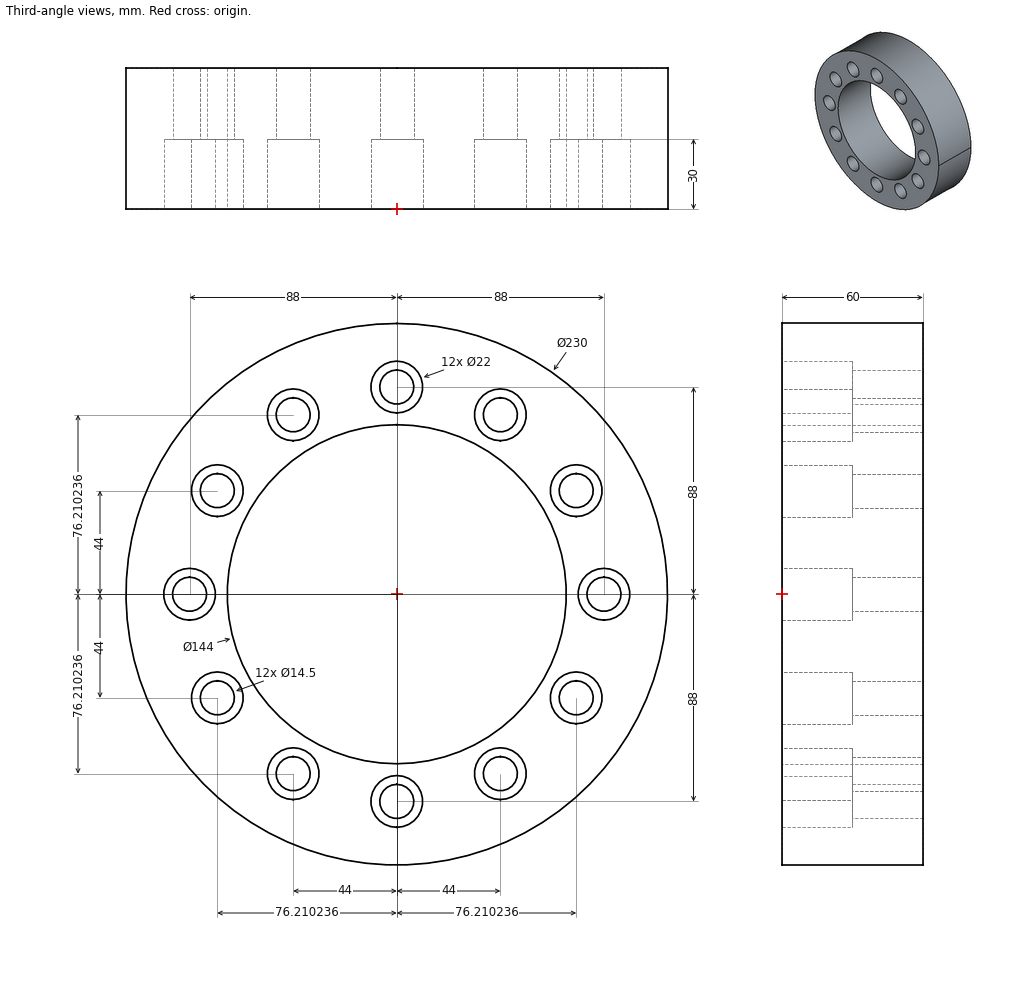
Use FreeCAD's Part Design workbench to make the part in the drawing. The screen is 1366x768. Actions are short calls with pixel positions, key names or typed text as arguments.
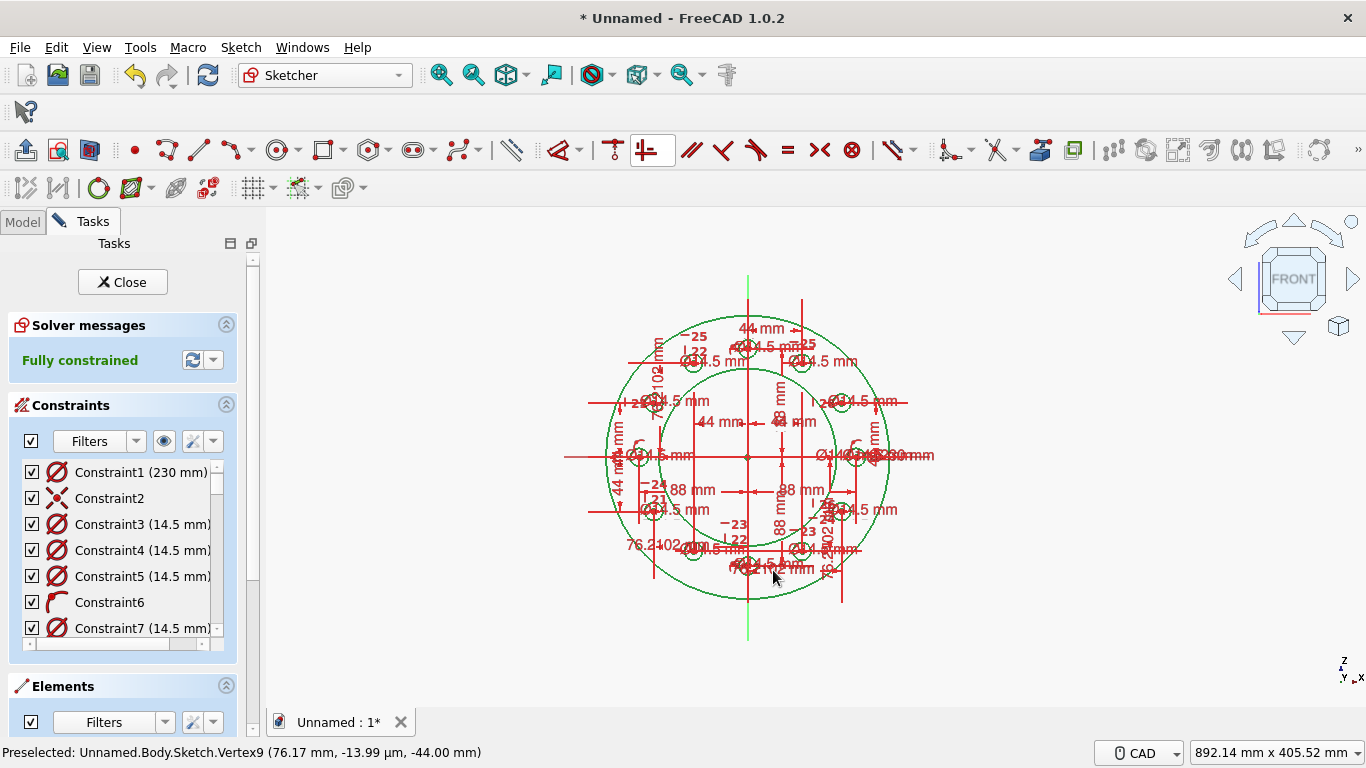
click(123, 282)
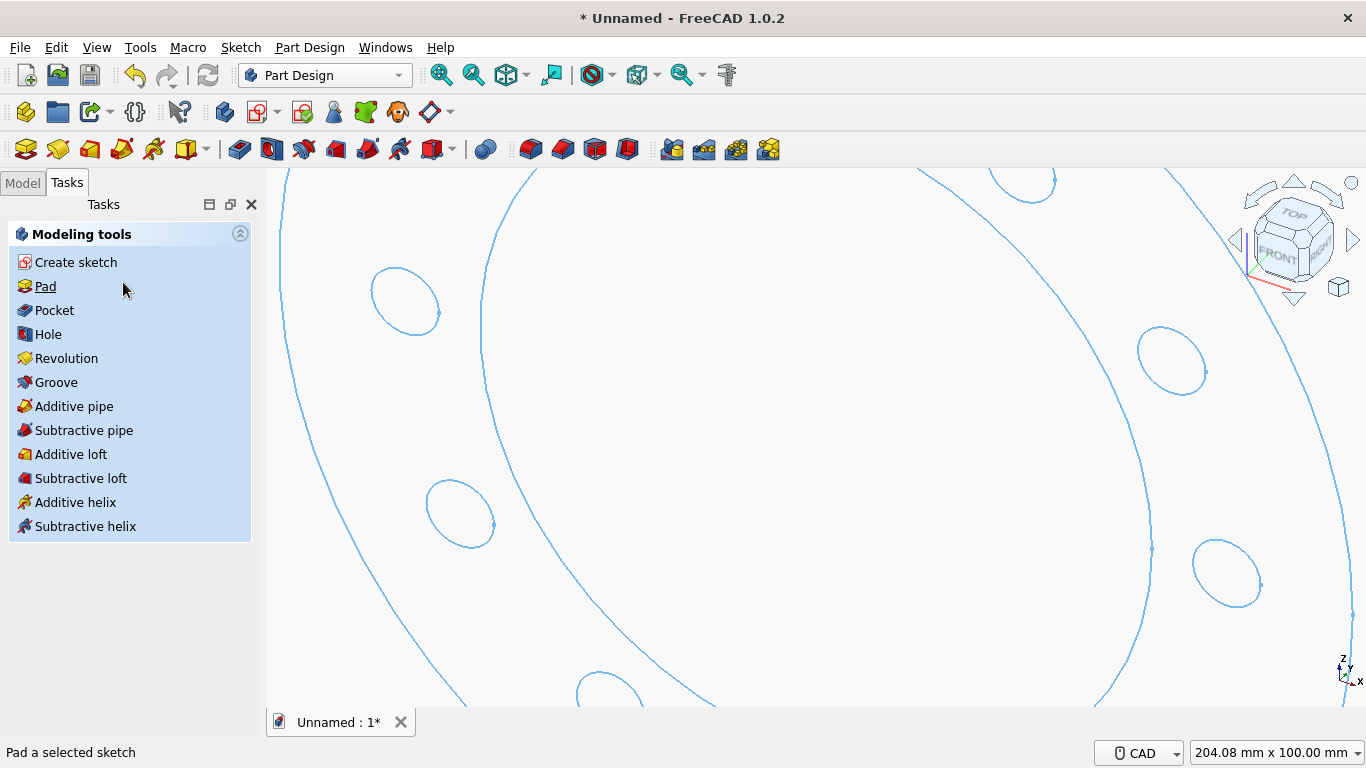
click(26, 150)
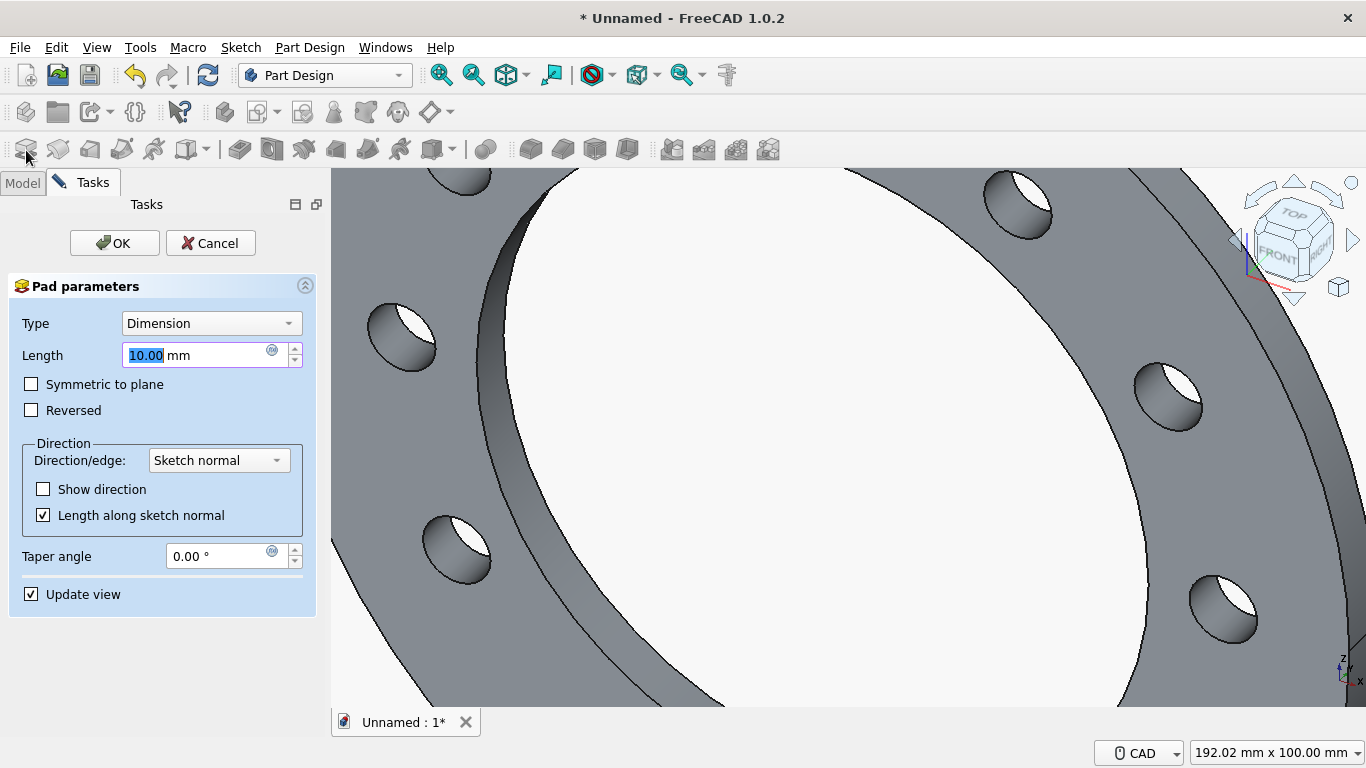
text(60)
key(Tab)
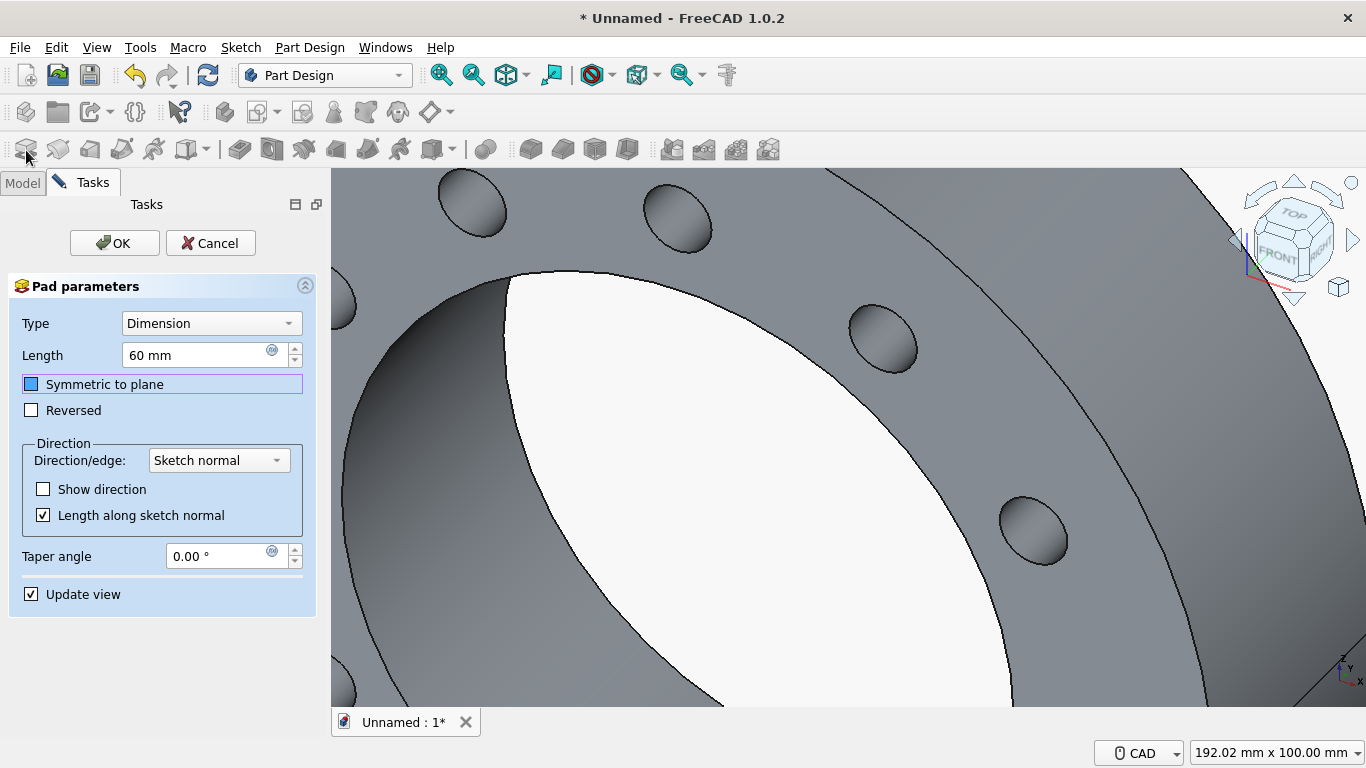
click(30, 410)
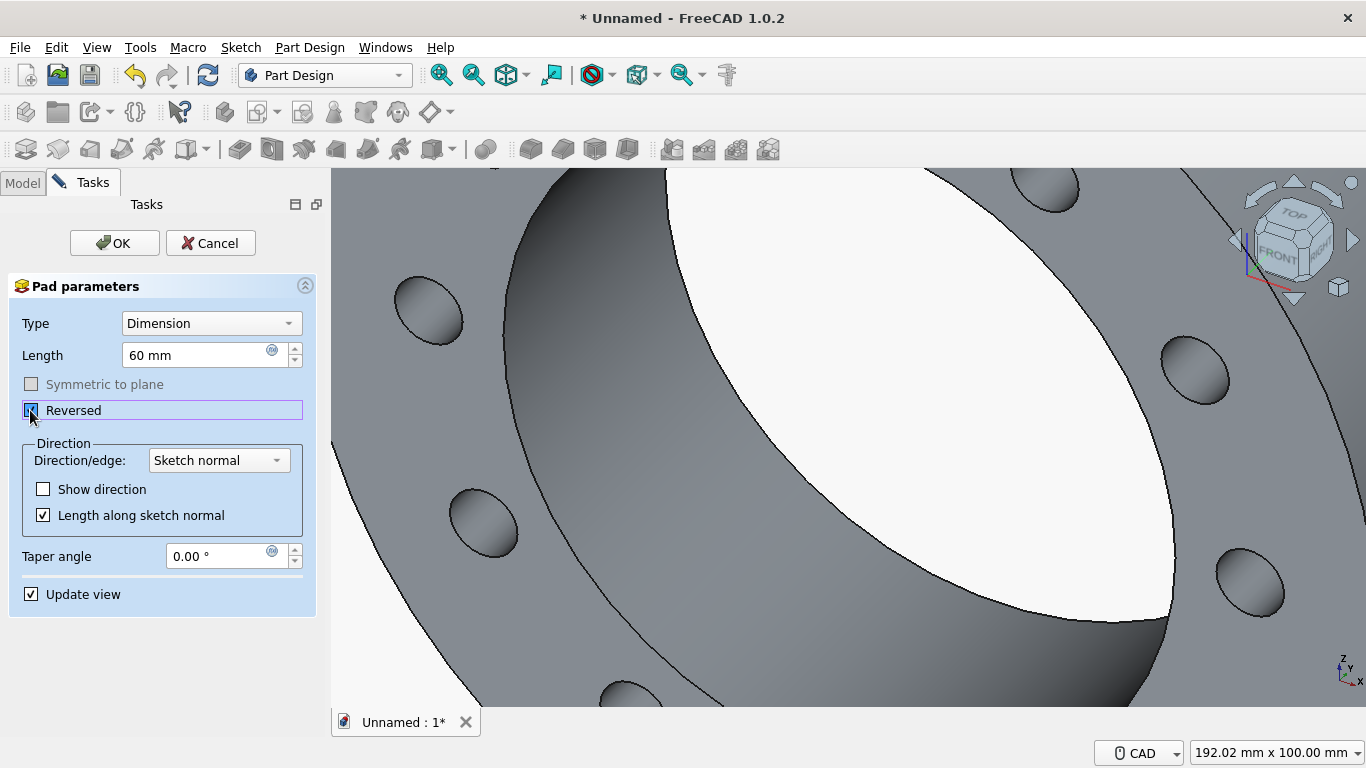
click(115, 243)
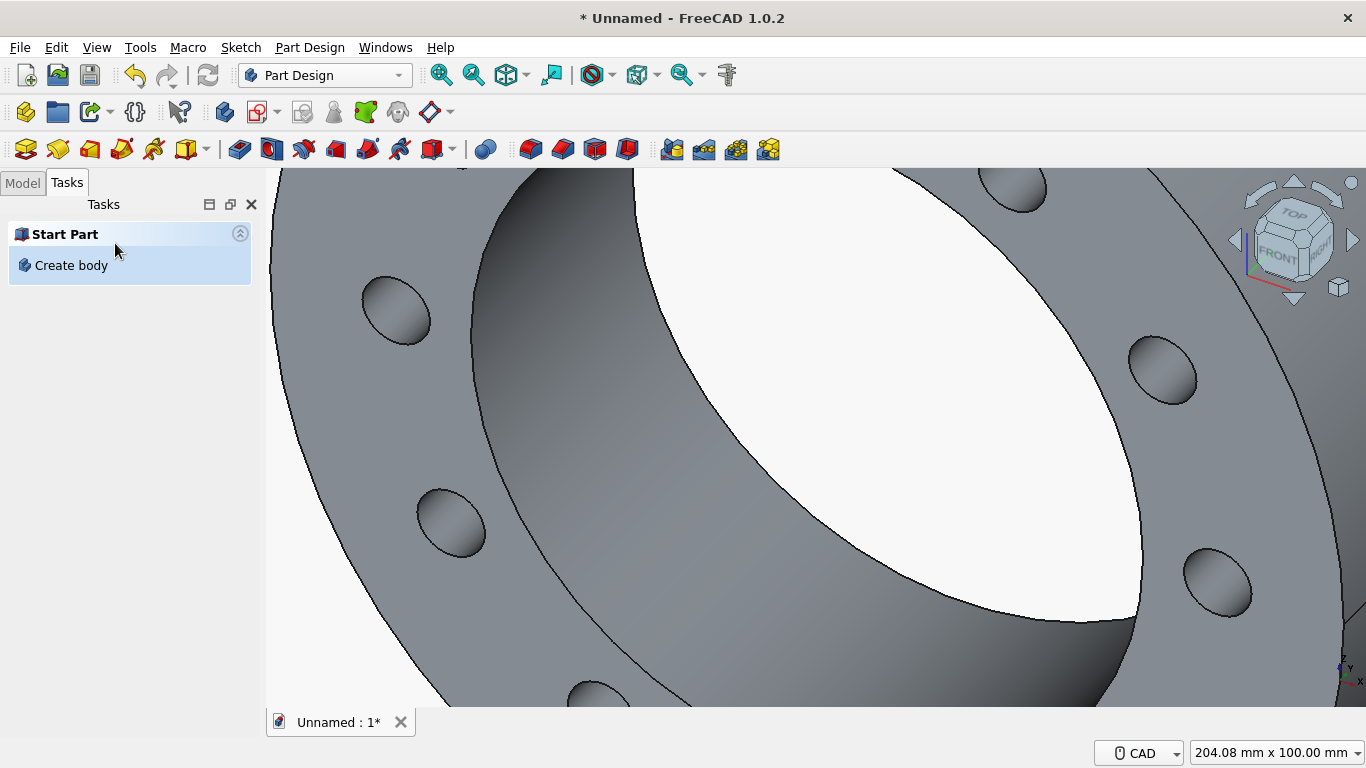
click(442, 76)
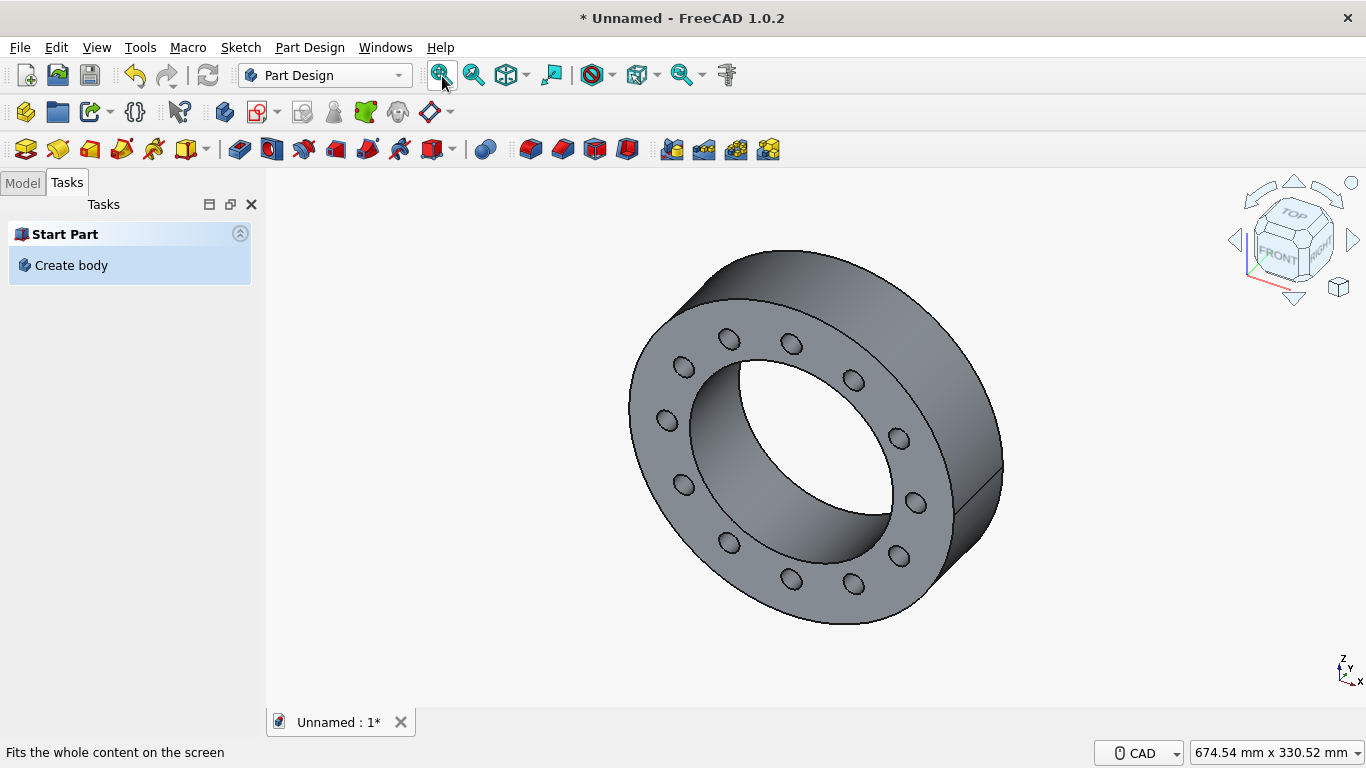
click(884, 404)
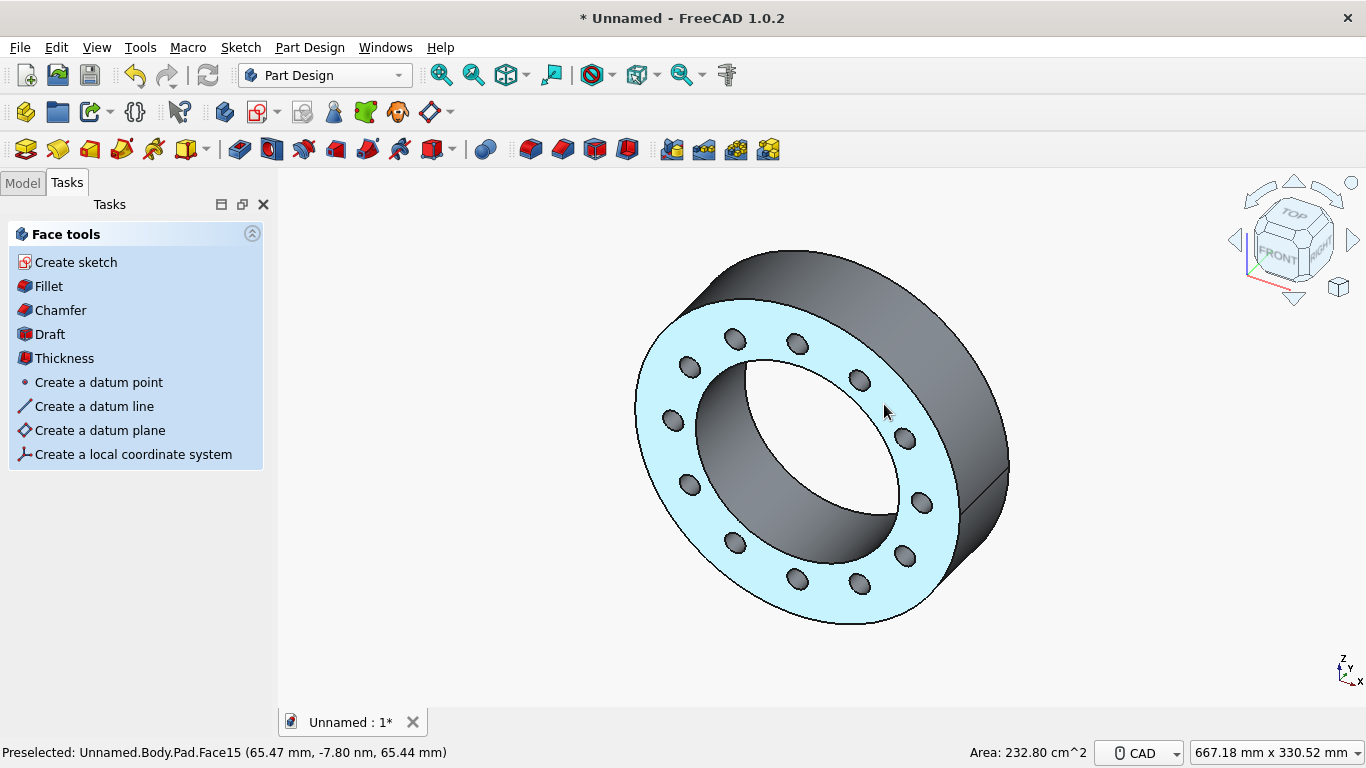
click(258, 112)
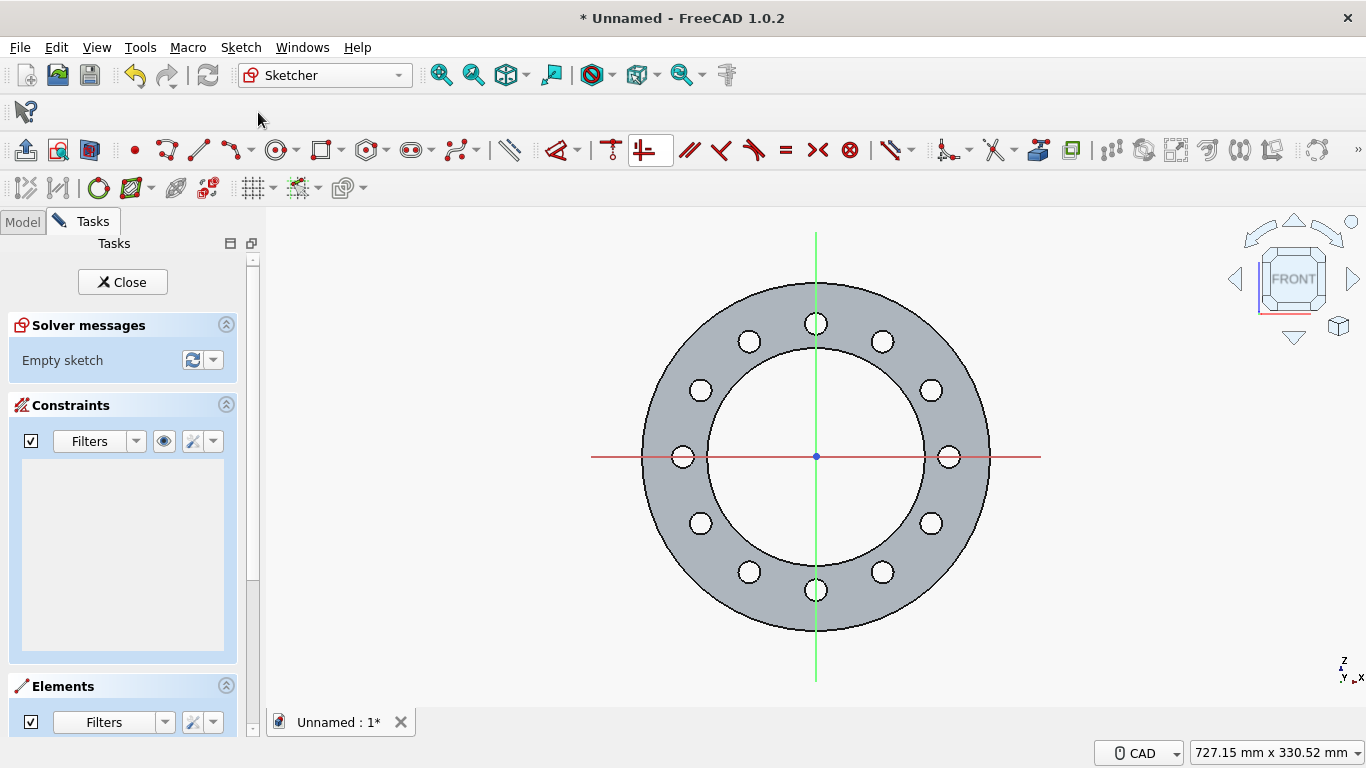
click(276, 150)